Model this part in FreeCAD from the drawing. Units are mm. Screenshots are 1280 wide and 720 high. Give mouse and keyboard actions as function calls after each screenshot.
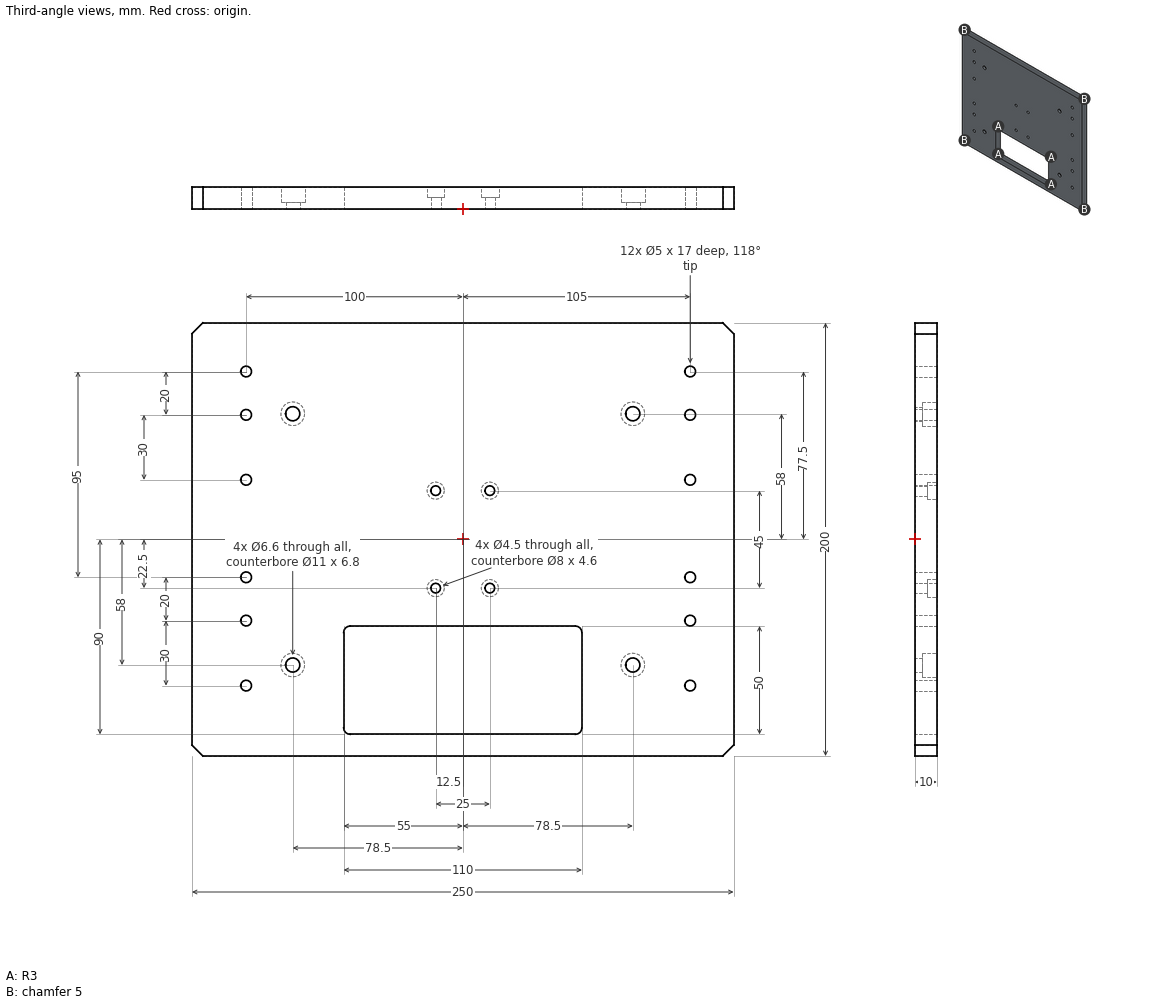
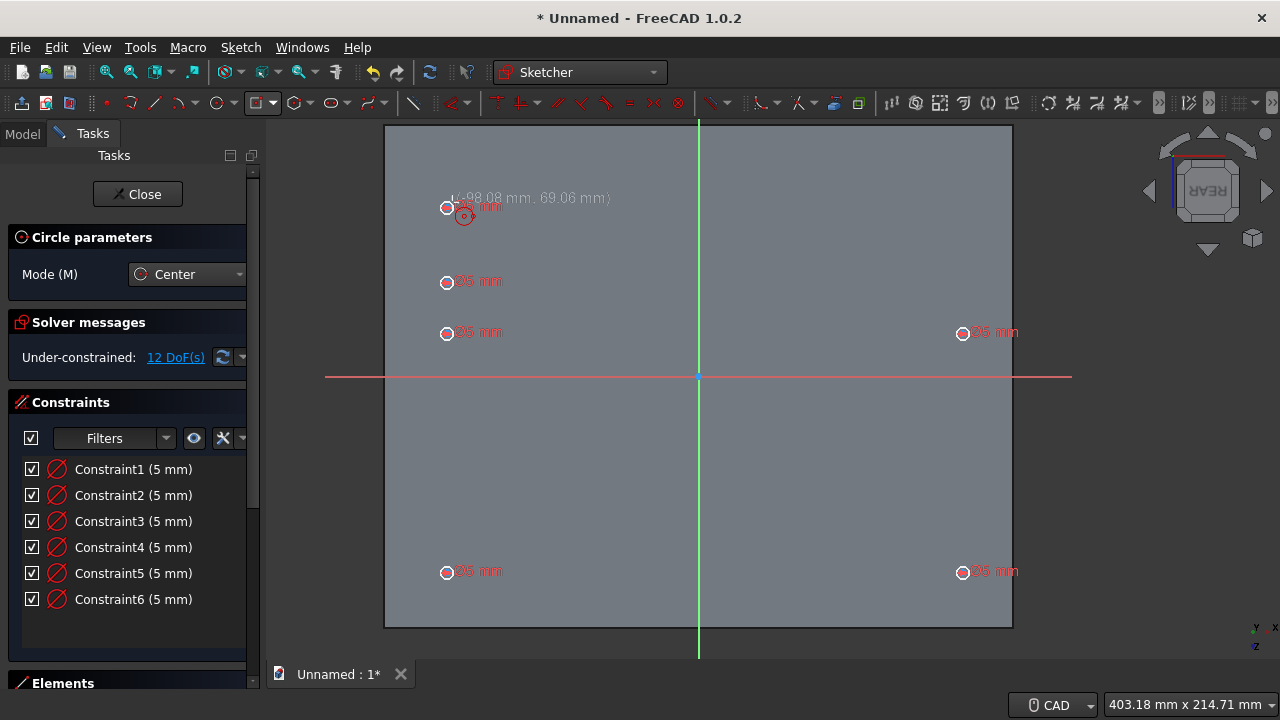
scroll(963, 282, up, 7)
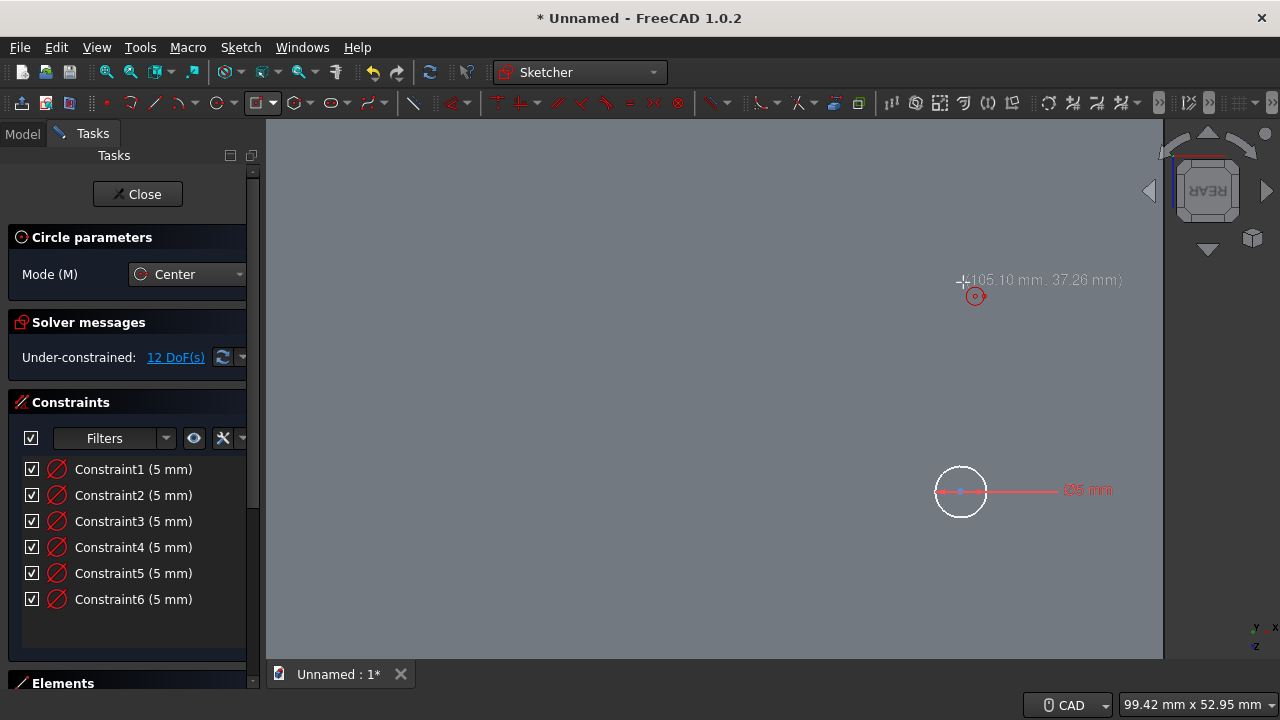
scroll(963, 282, down, 7)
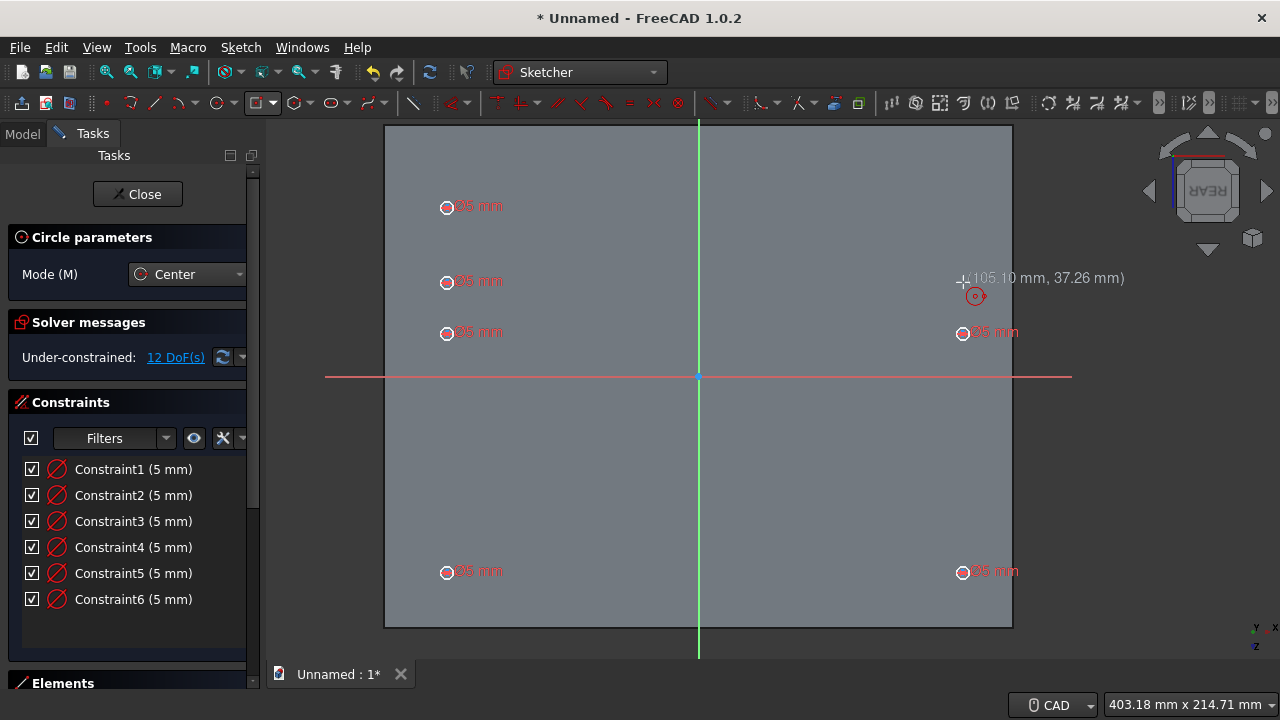
click(963, 282)
move(967, 278)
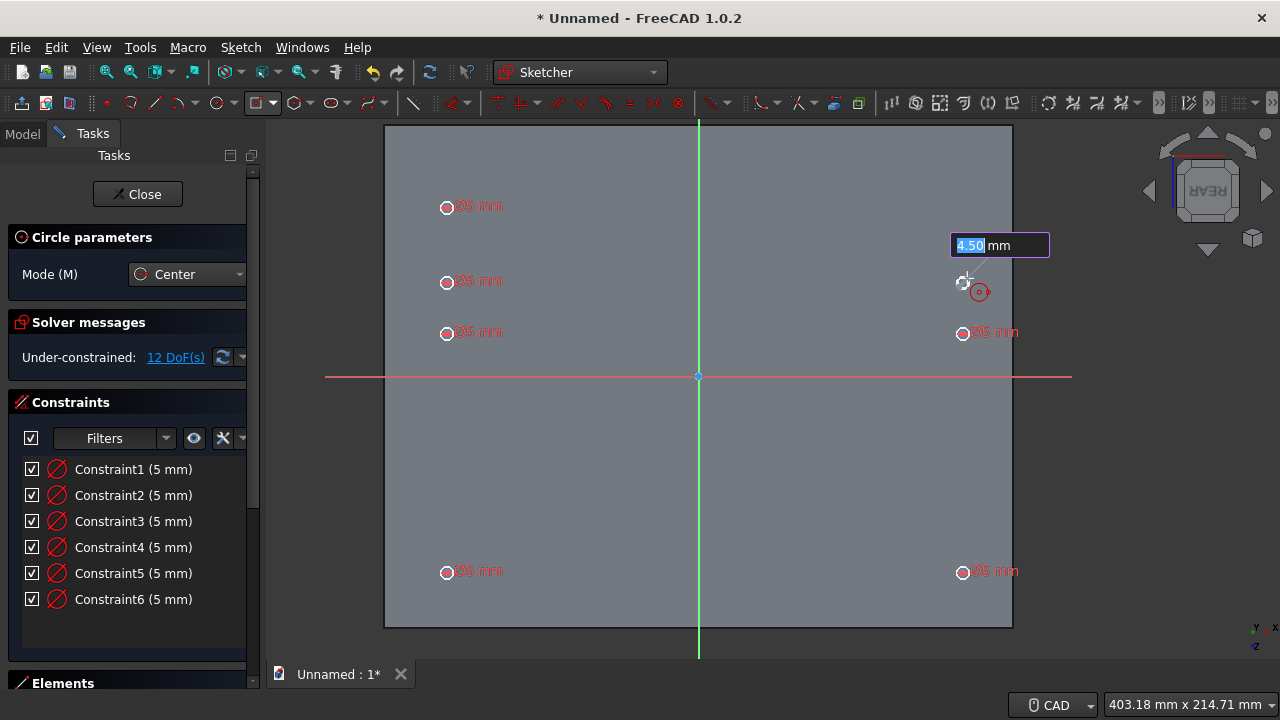
text(5)
key(Return)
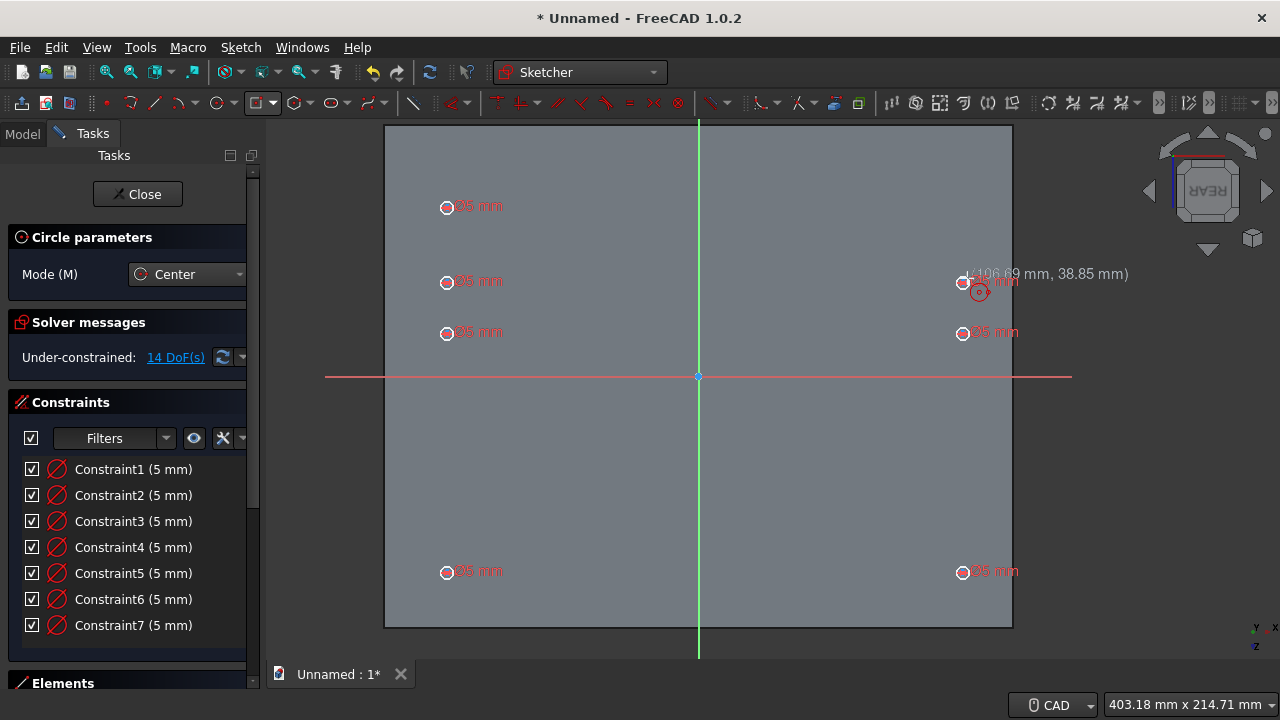
scroll(963, 207, up, 7)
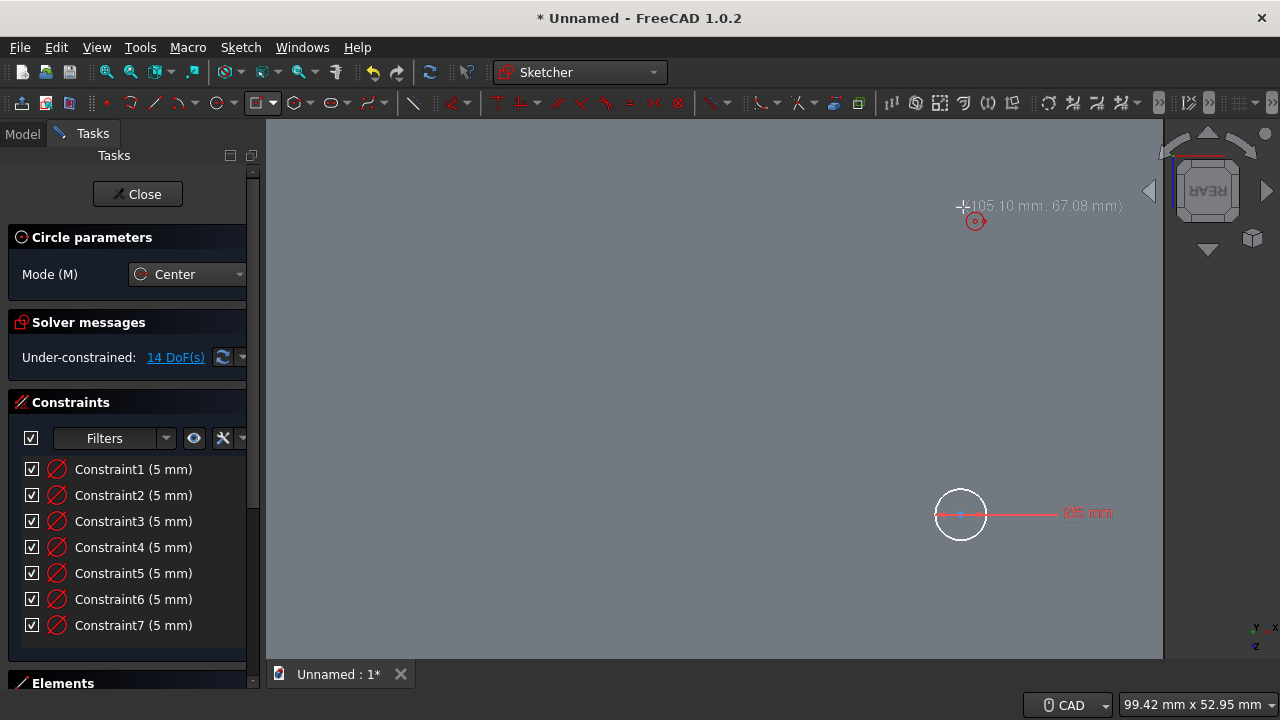
scroll(963, 207, down, 7)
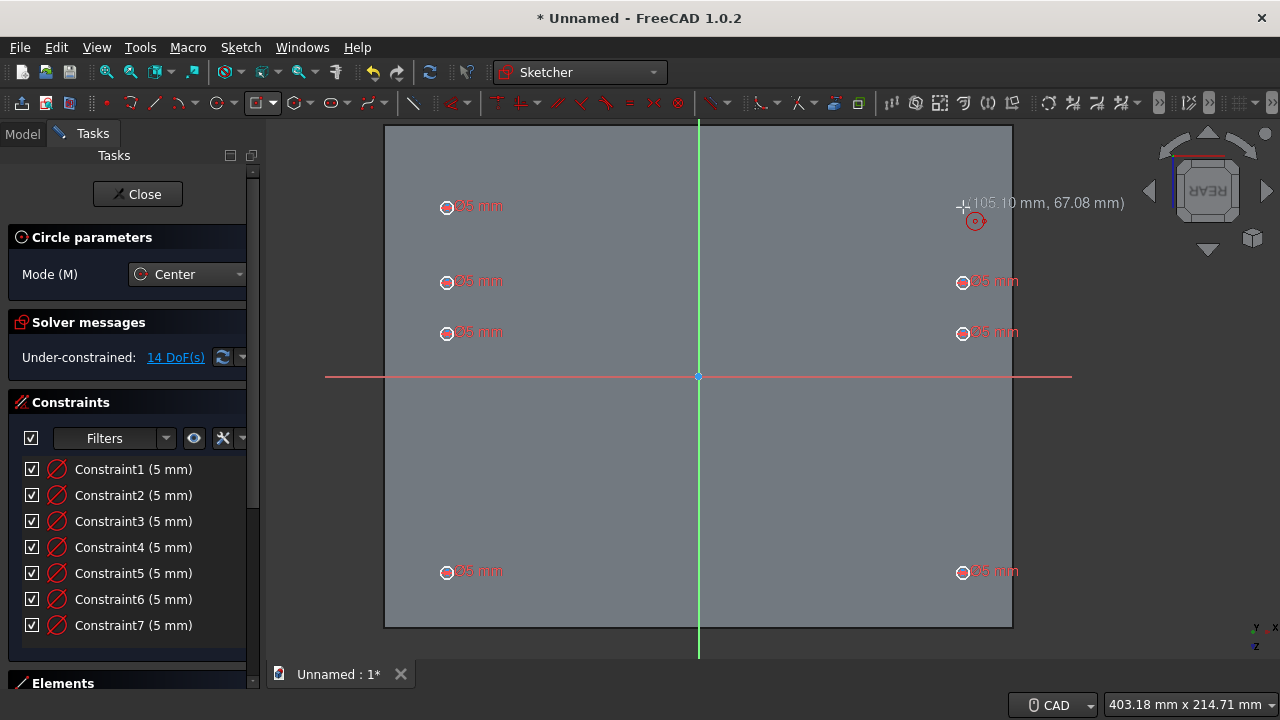
click(963, 207)
move(967, 202)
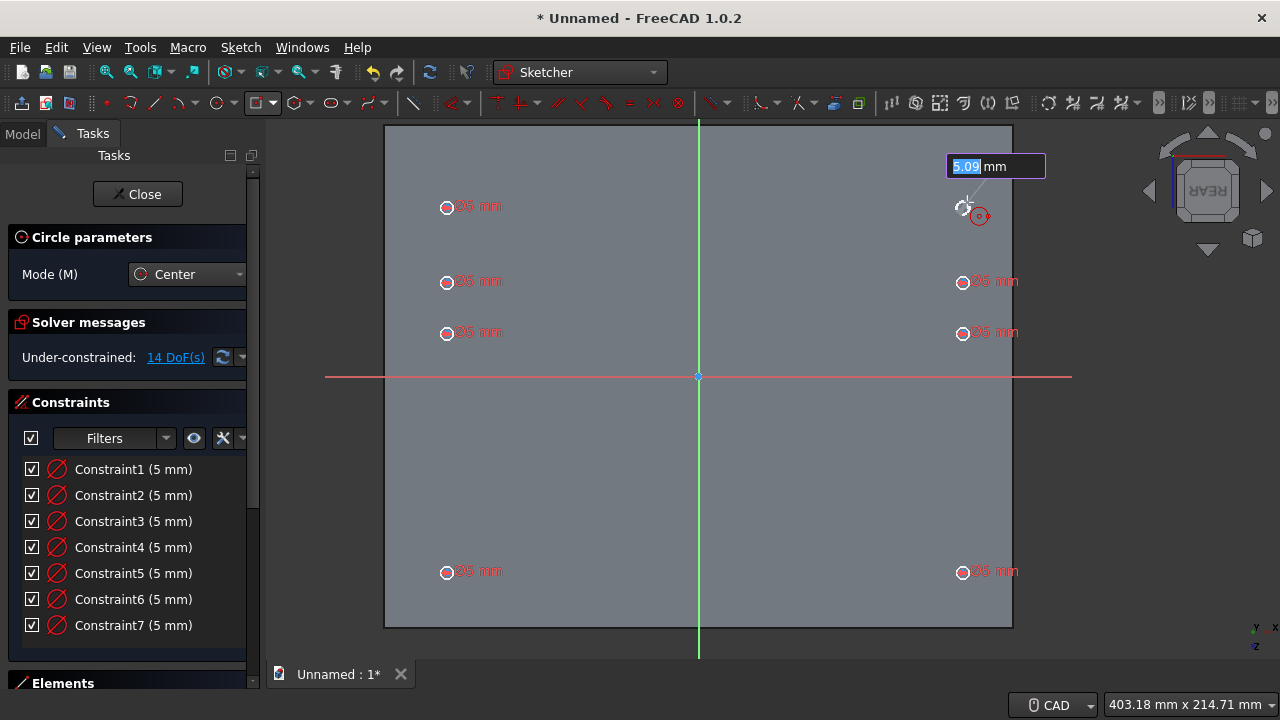
text(5)
key(Return)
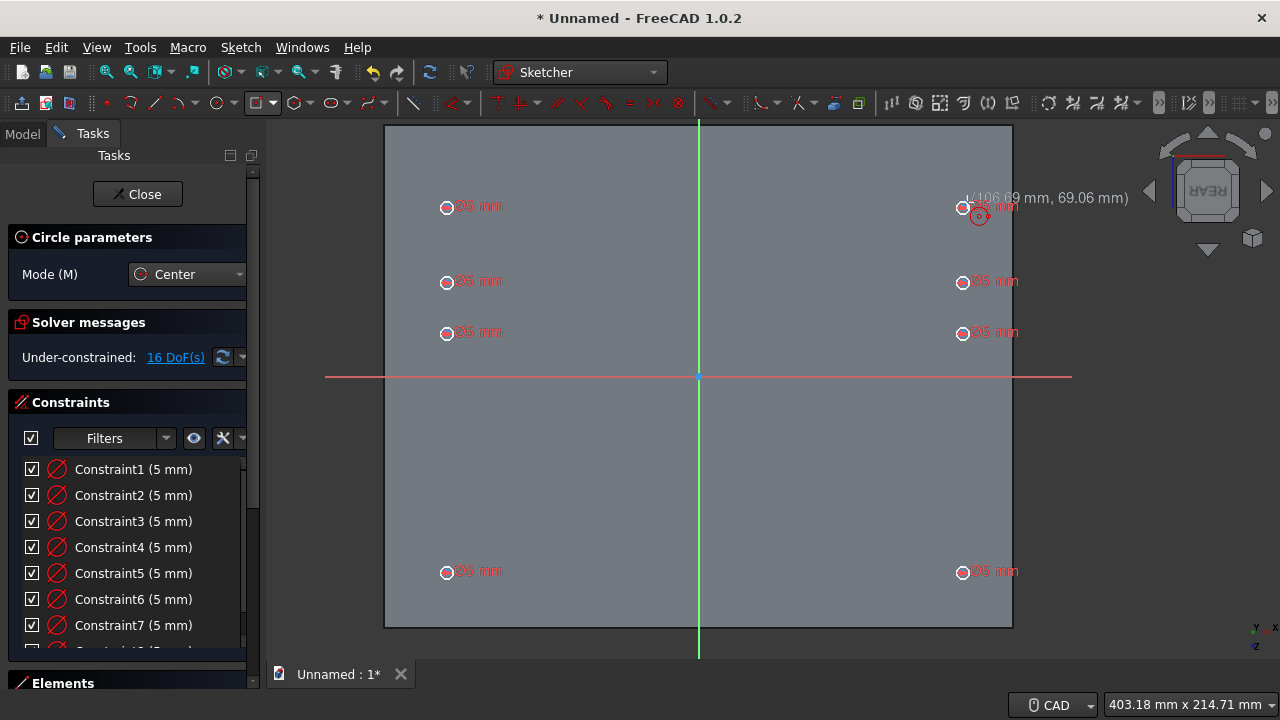
scroll(447, 521, up, 7)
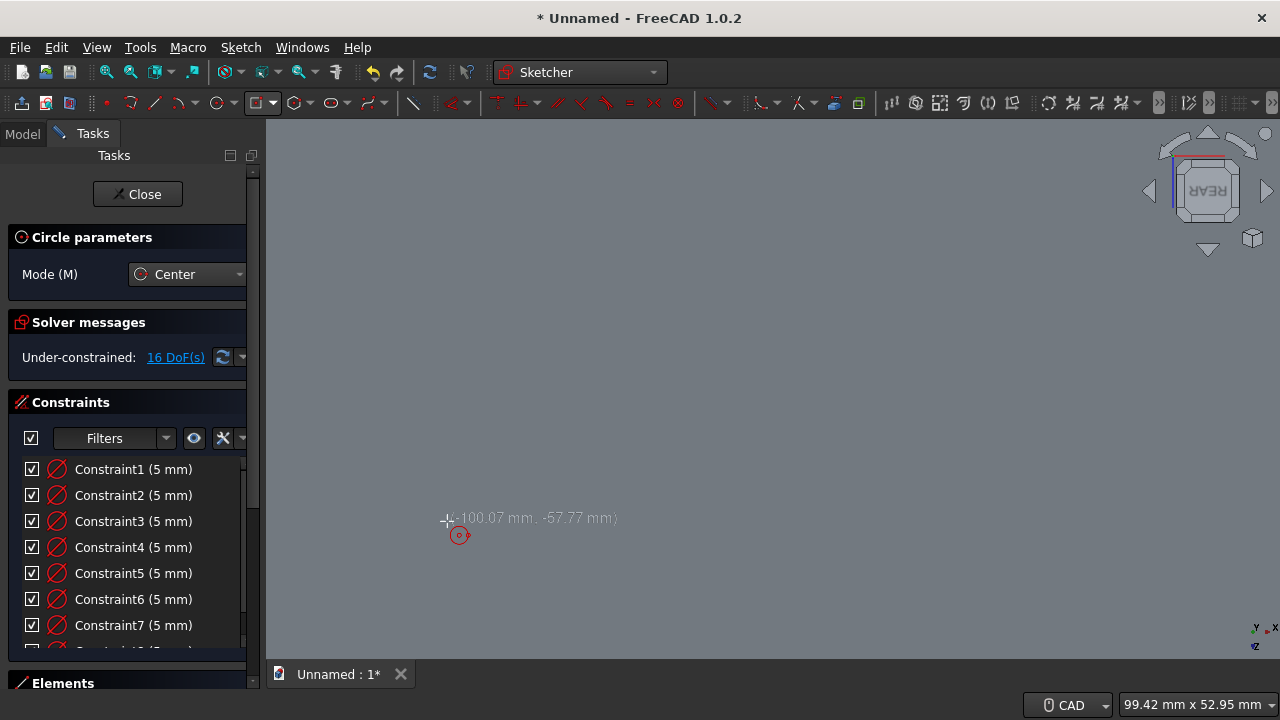
scroll(447, 521, down, 7)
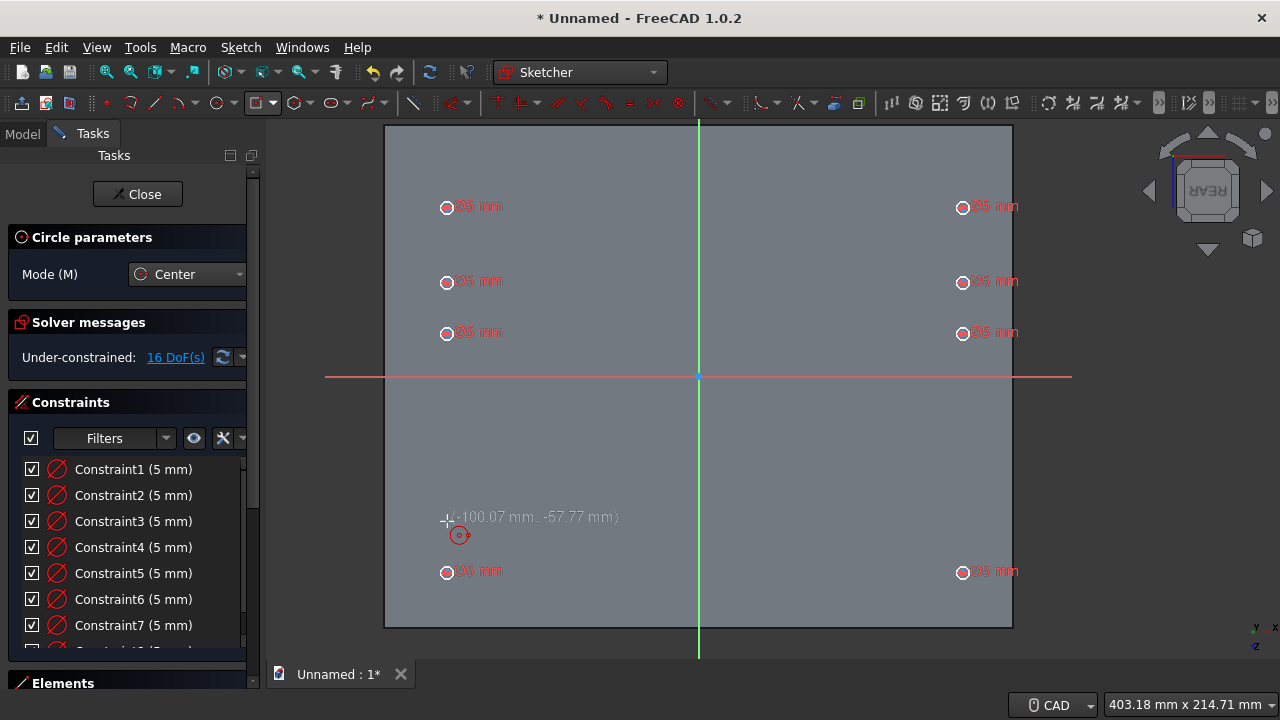
click(447, 521)
move(452, 517)